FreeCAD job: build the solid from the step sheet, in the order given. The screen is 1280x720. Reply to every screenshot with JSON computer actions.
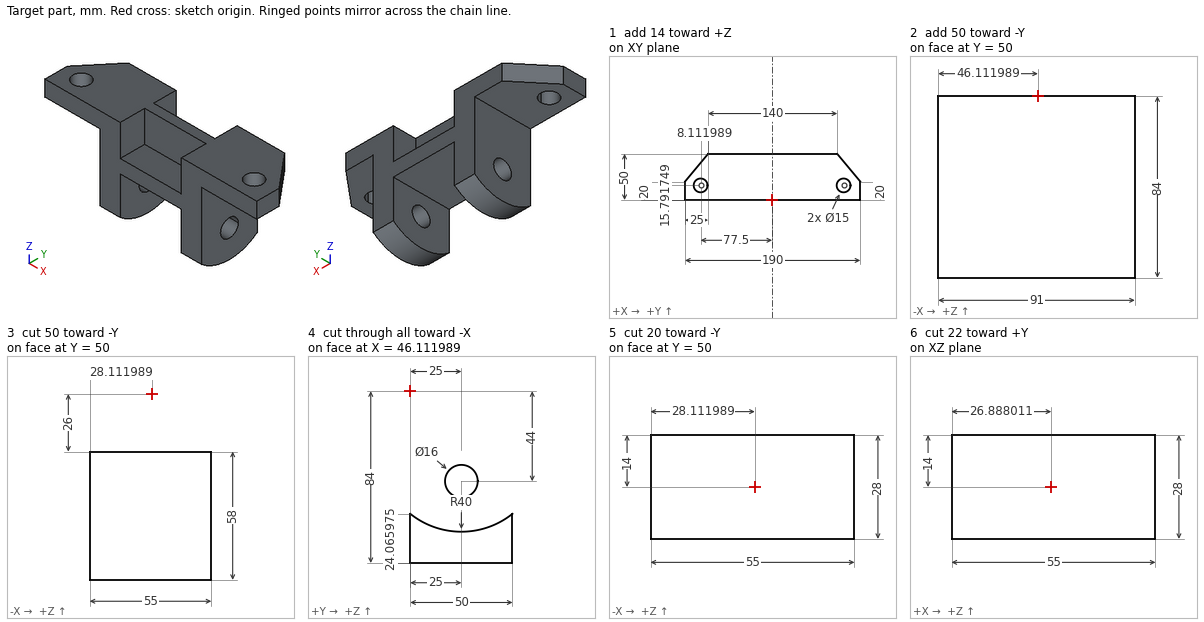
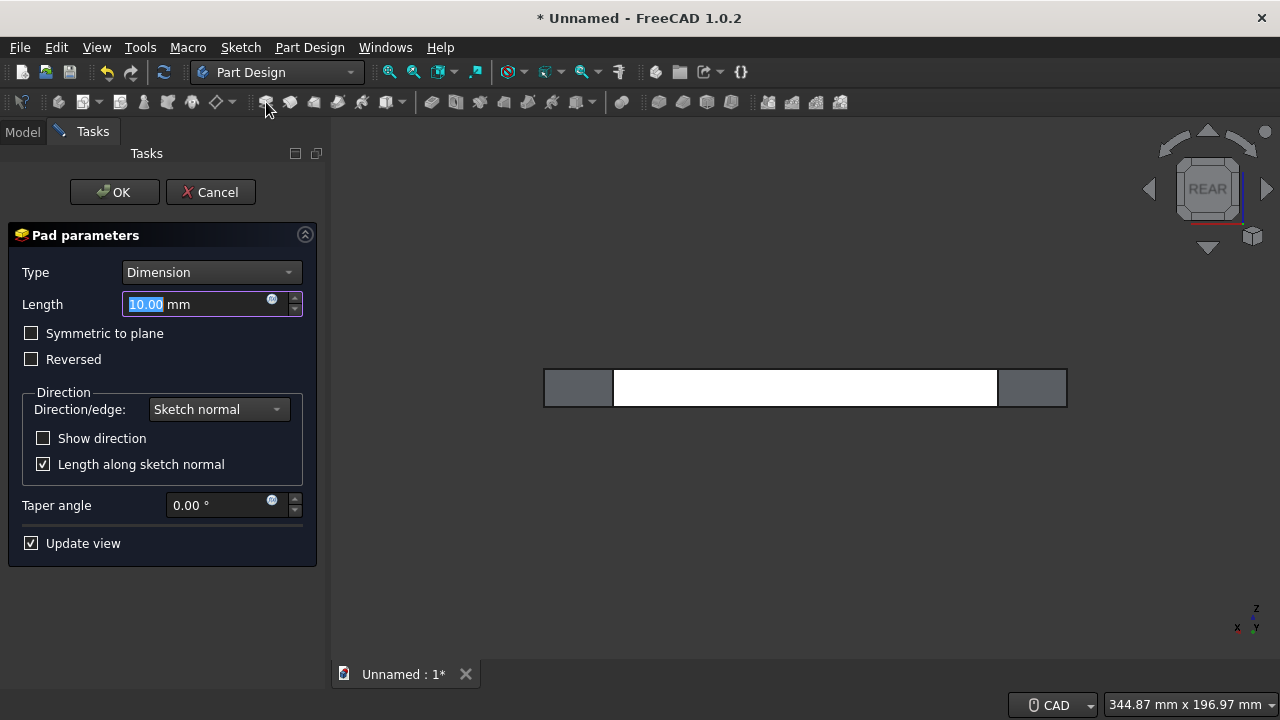
{"action": "type", "text": "50"}
{"action": "key", "text": "Tab"}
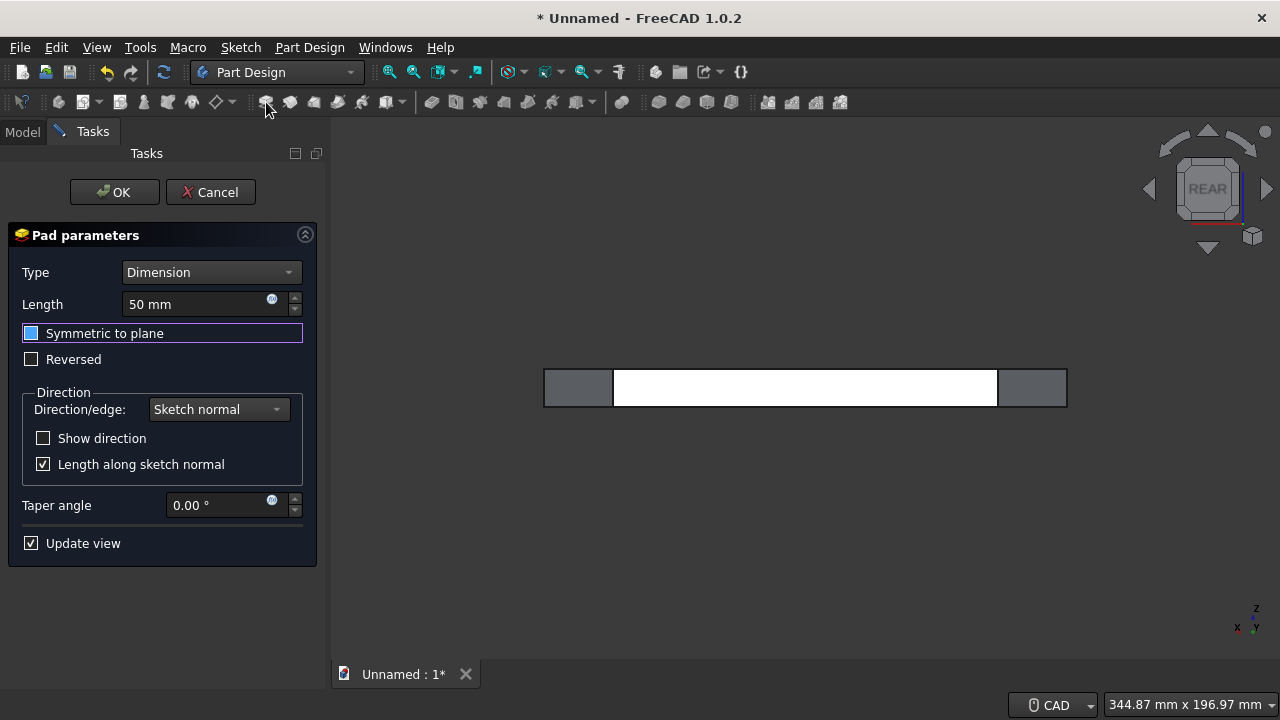
{"action": "left_click", "coordinate": [30, 359]}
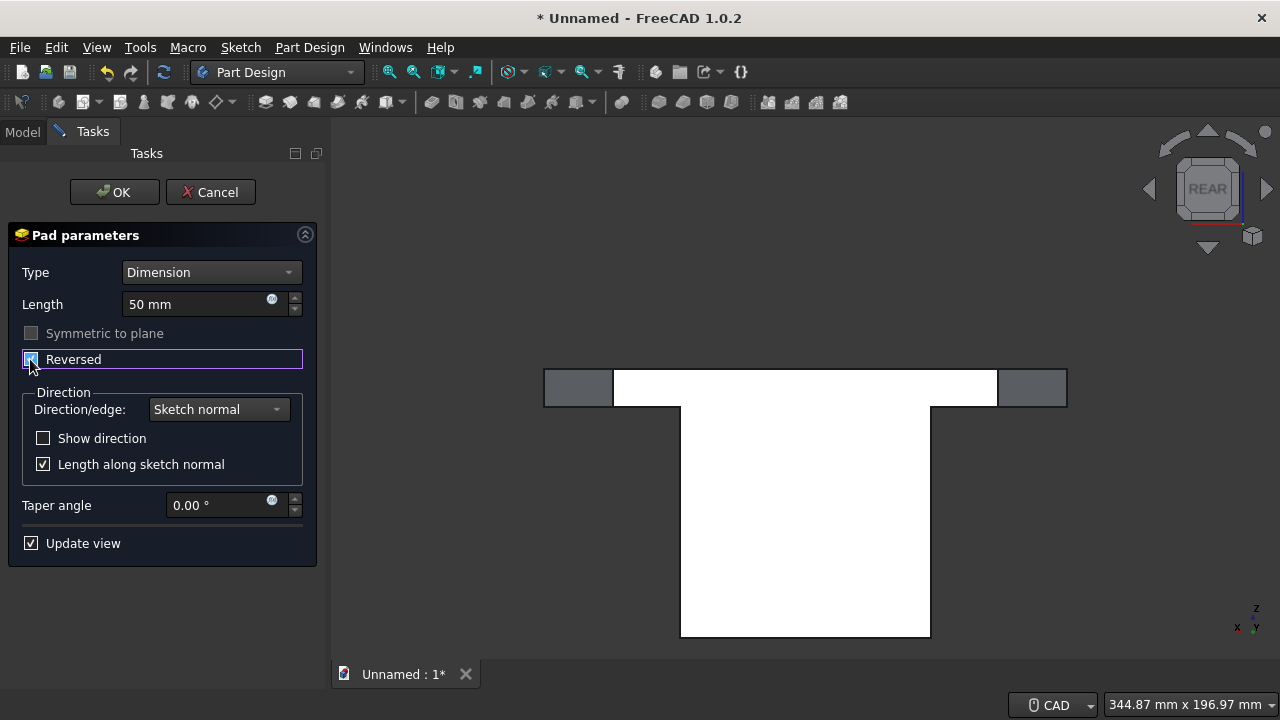
{"action": "left_click", "coordinate": [115, 192]}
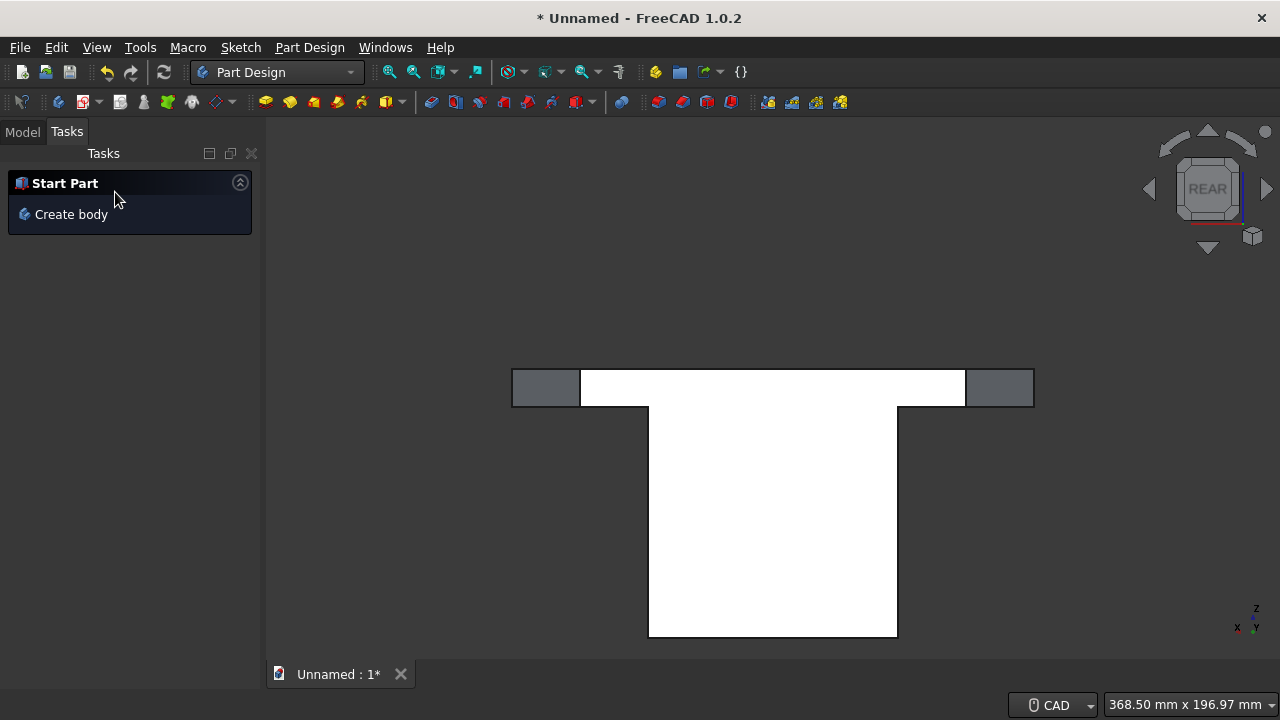
{"action": "left_click", "coordinate": [773, 503]}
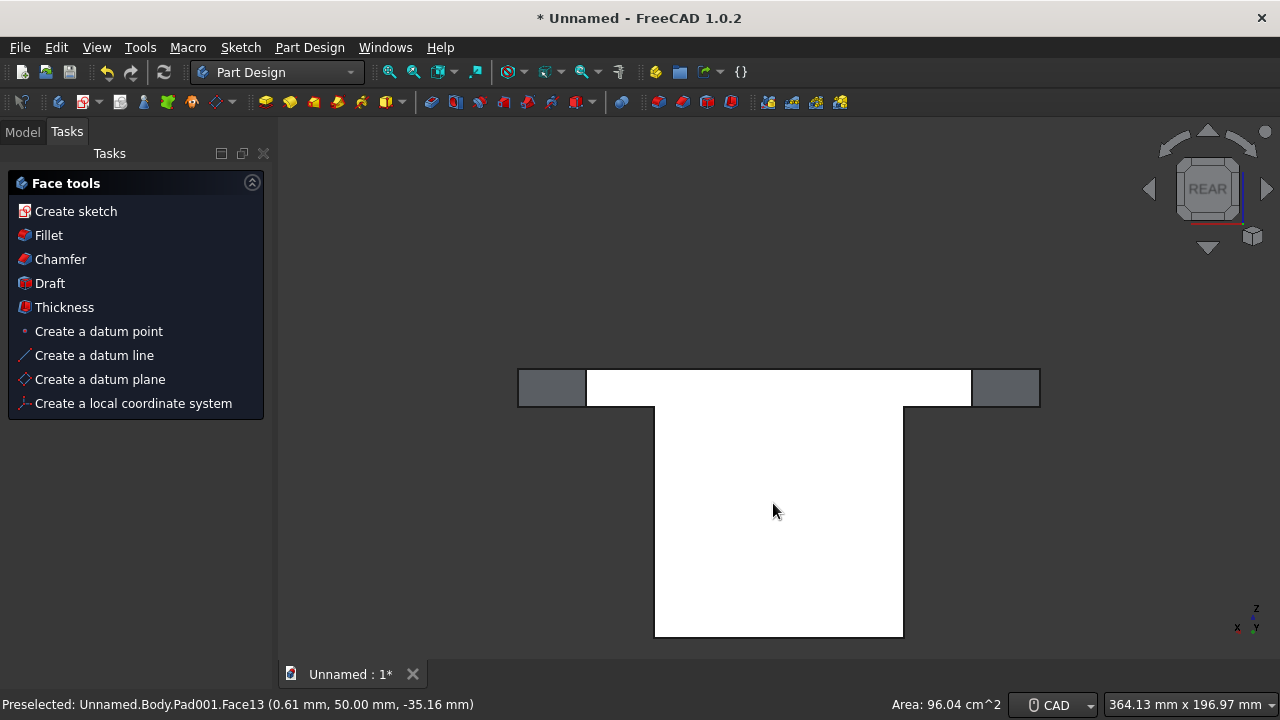
{"action": "left_click", "coordinate": [84, 102]}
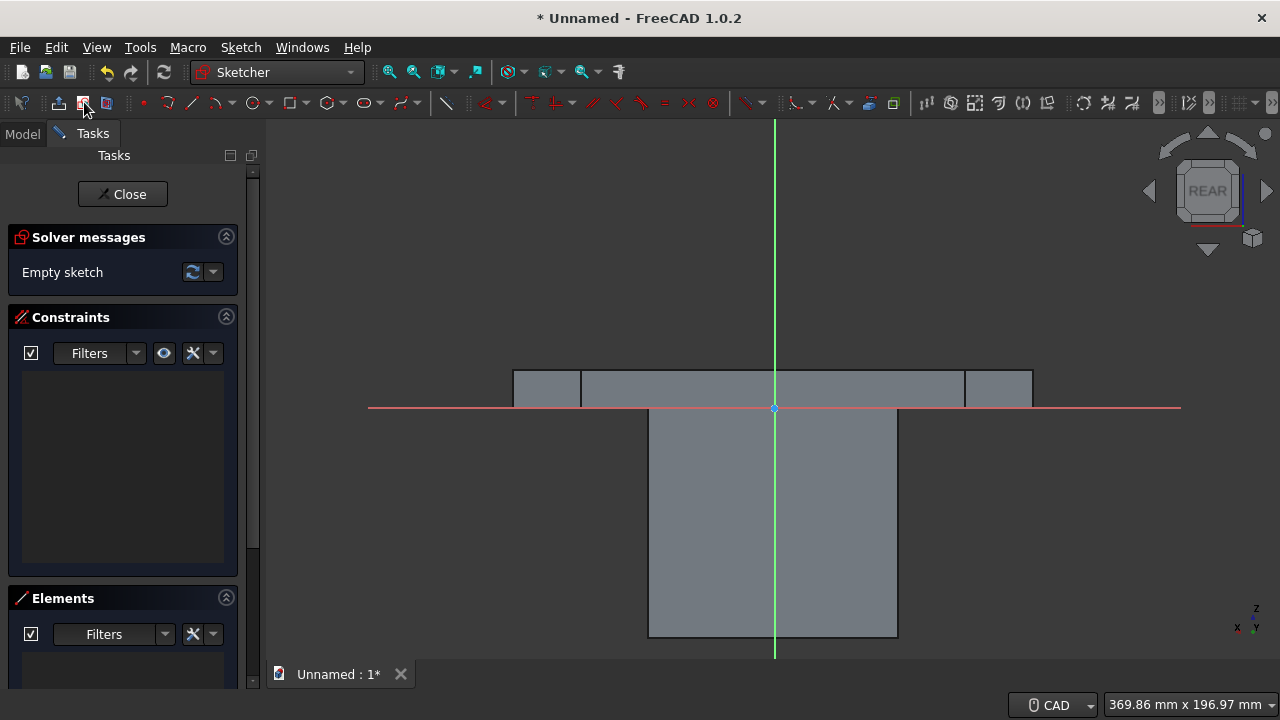
{"action": "scroll", "coordinate": [395, 147], "scroll_direction": "down", "scroll_amount": 1}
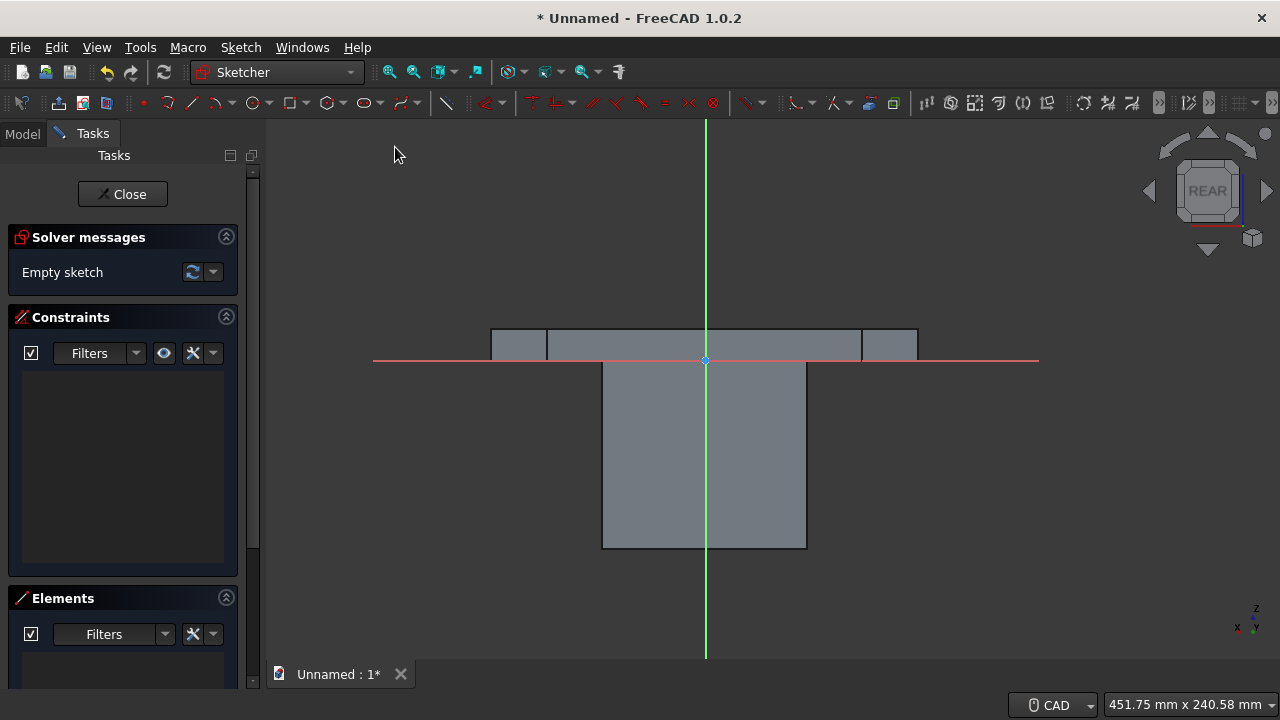
{"action": "scroll", "coordinate": [705, 536], "scroll_direction": "up", "scroll_amount": 3}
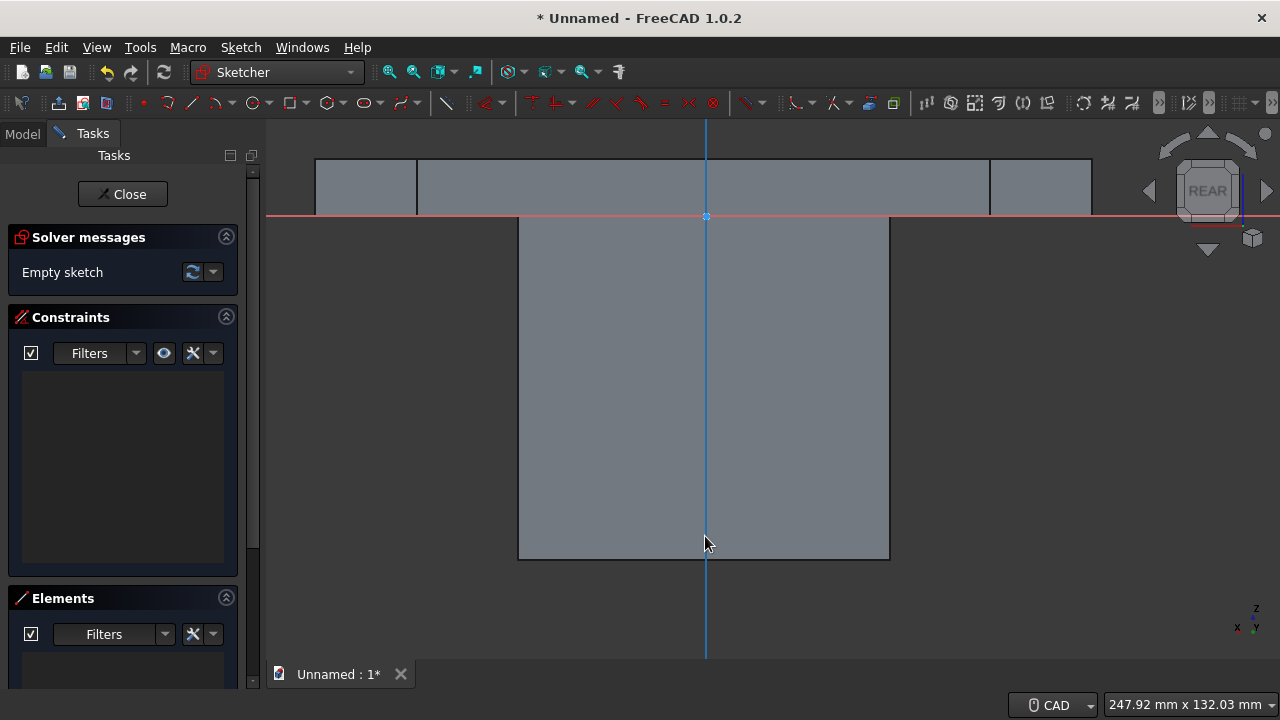
{"action": "left_click", "coordinate": [290, 104]}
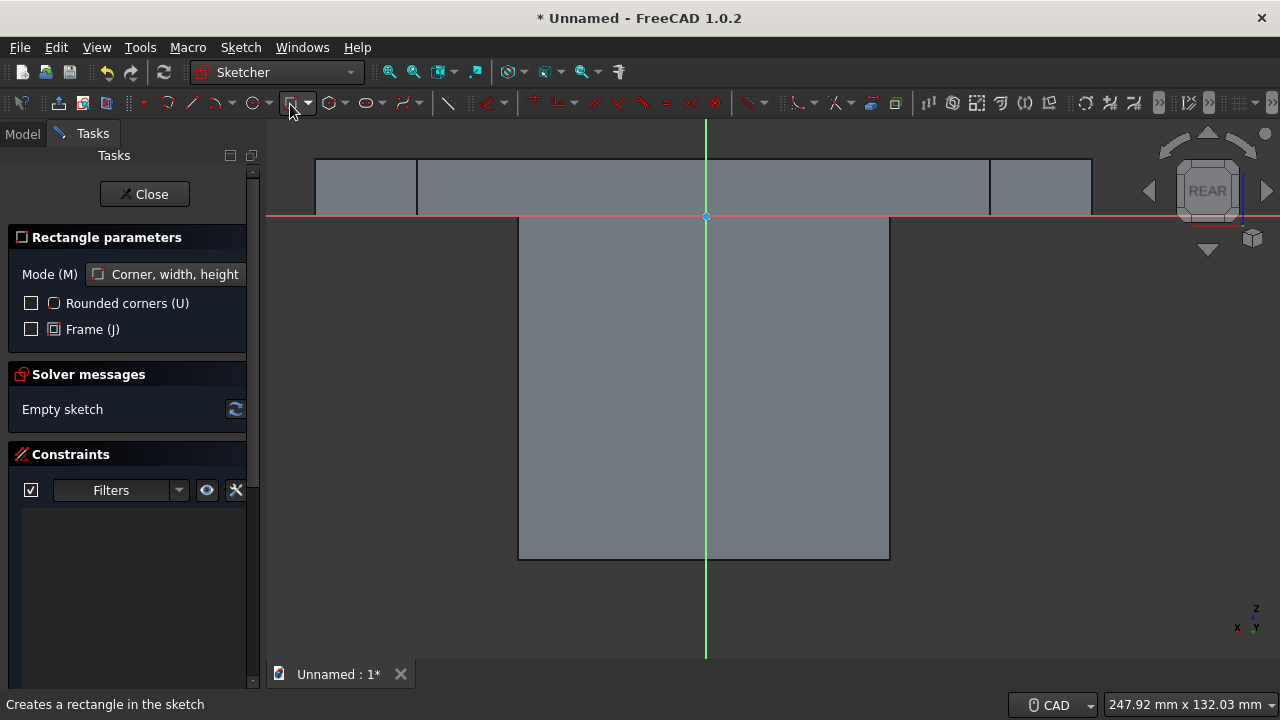
{"action": "left_click", "coordinate": [591, 323]}
{"action": "mouse_move", "coordinate": [816, 560]}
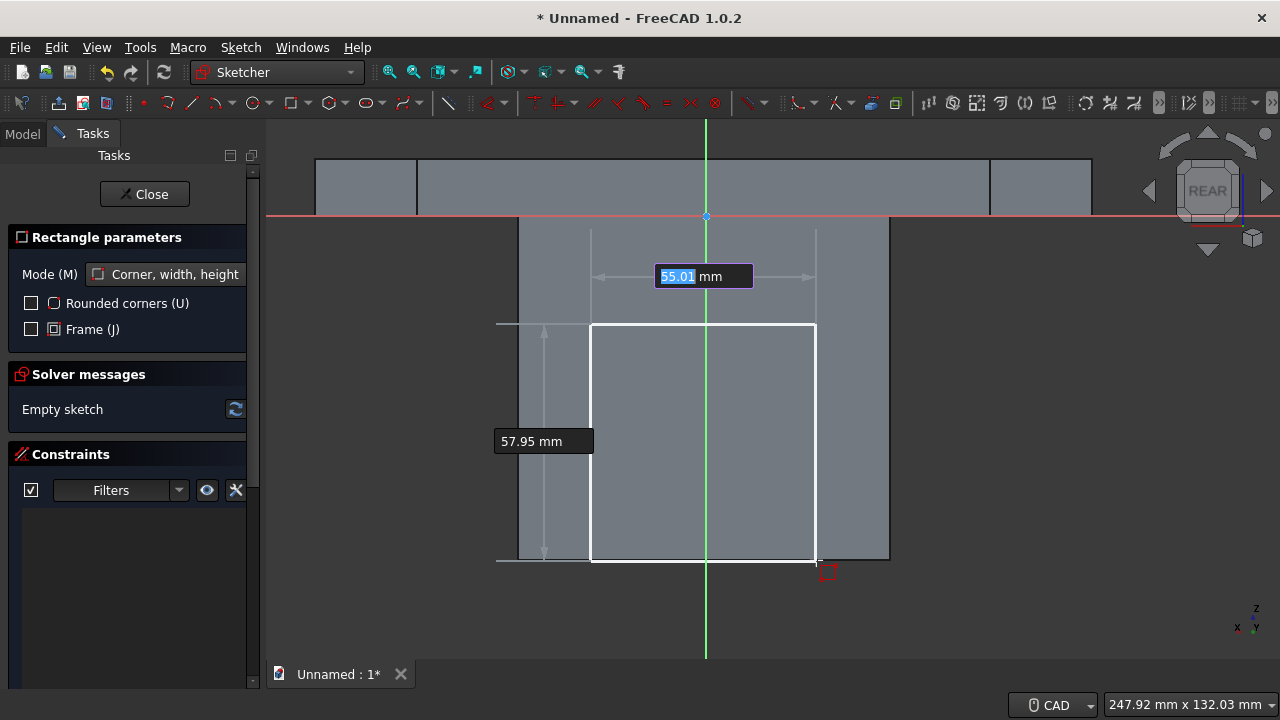
{"action": "type", "text": "55"}
{"action": "key", "text": "Tab"}
{"action": "type", "text": "58"}
{"action": "key", "text": "Return"}
{"action": "key", "text": "Escape"}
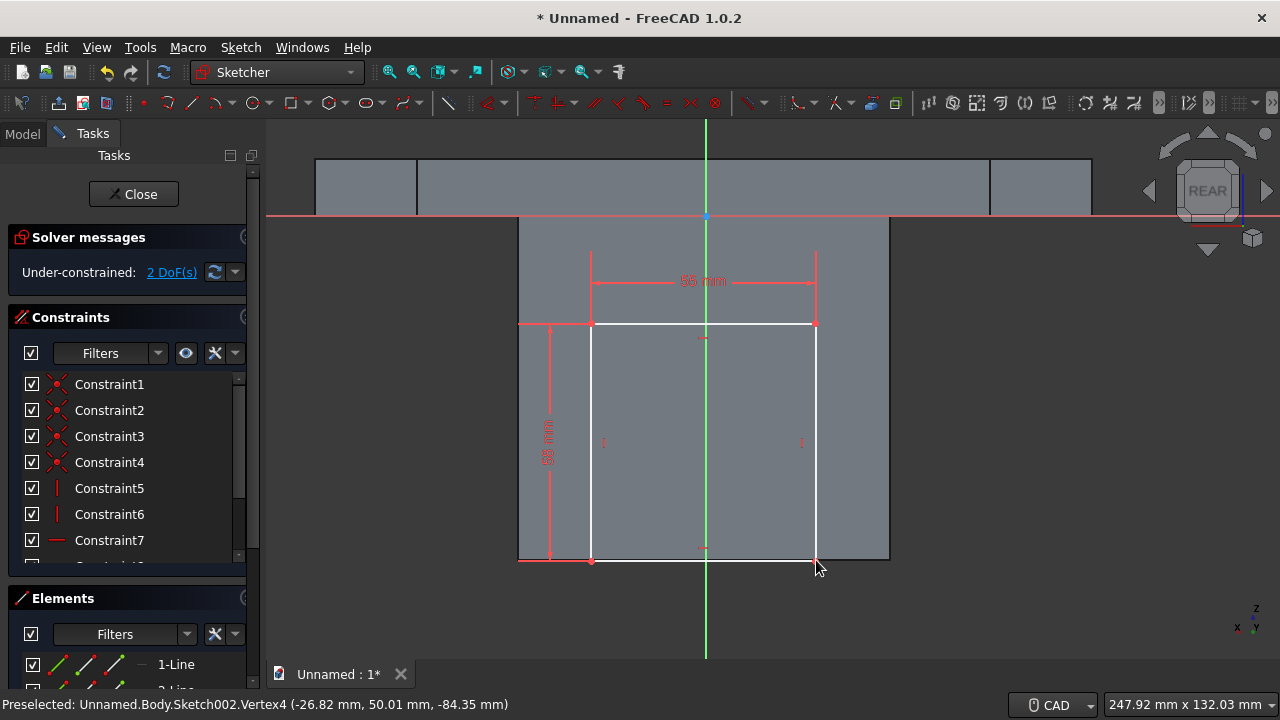
{"action": "left_click", "coordinate": [488, 104]}